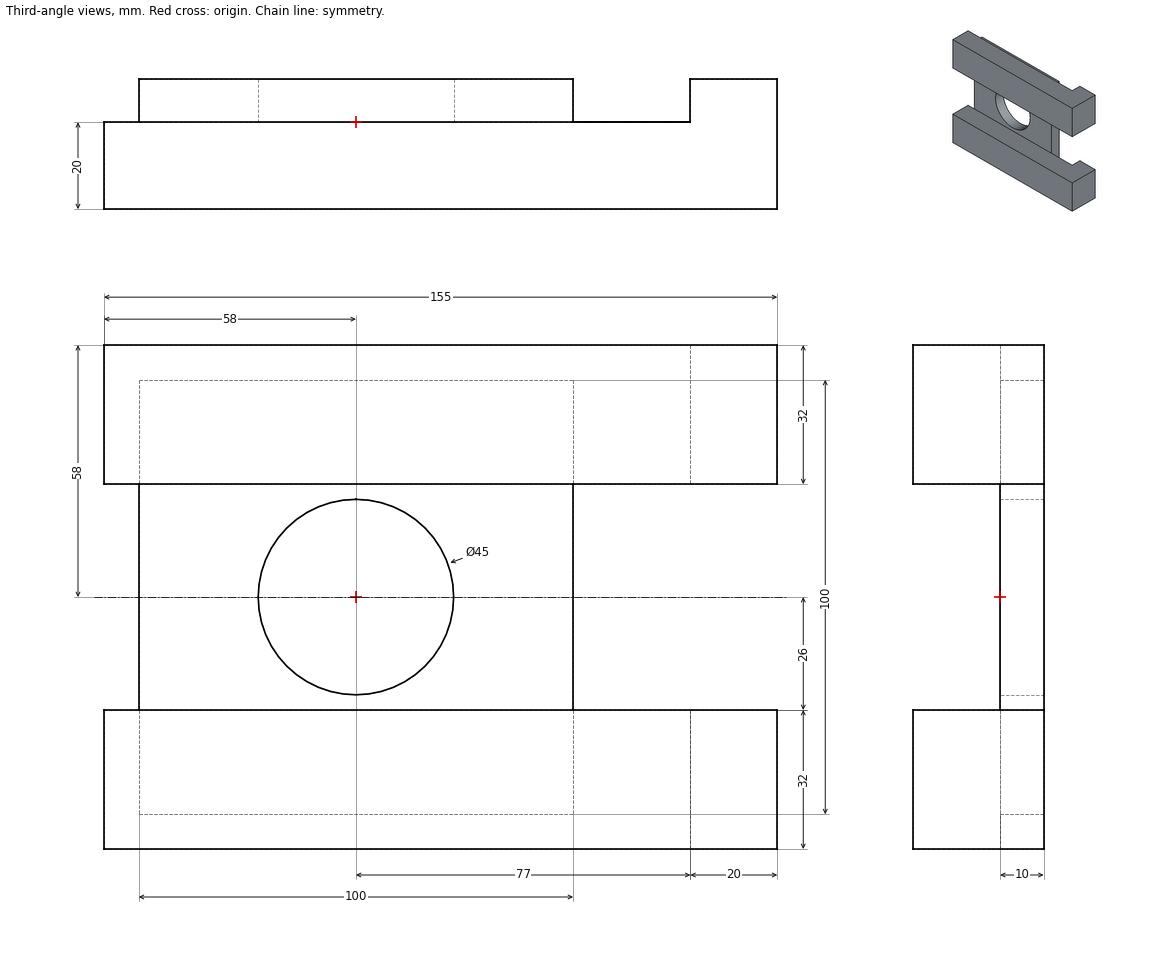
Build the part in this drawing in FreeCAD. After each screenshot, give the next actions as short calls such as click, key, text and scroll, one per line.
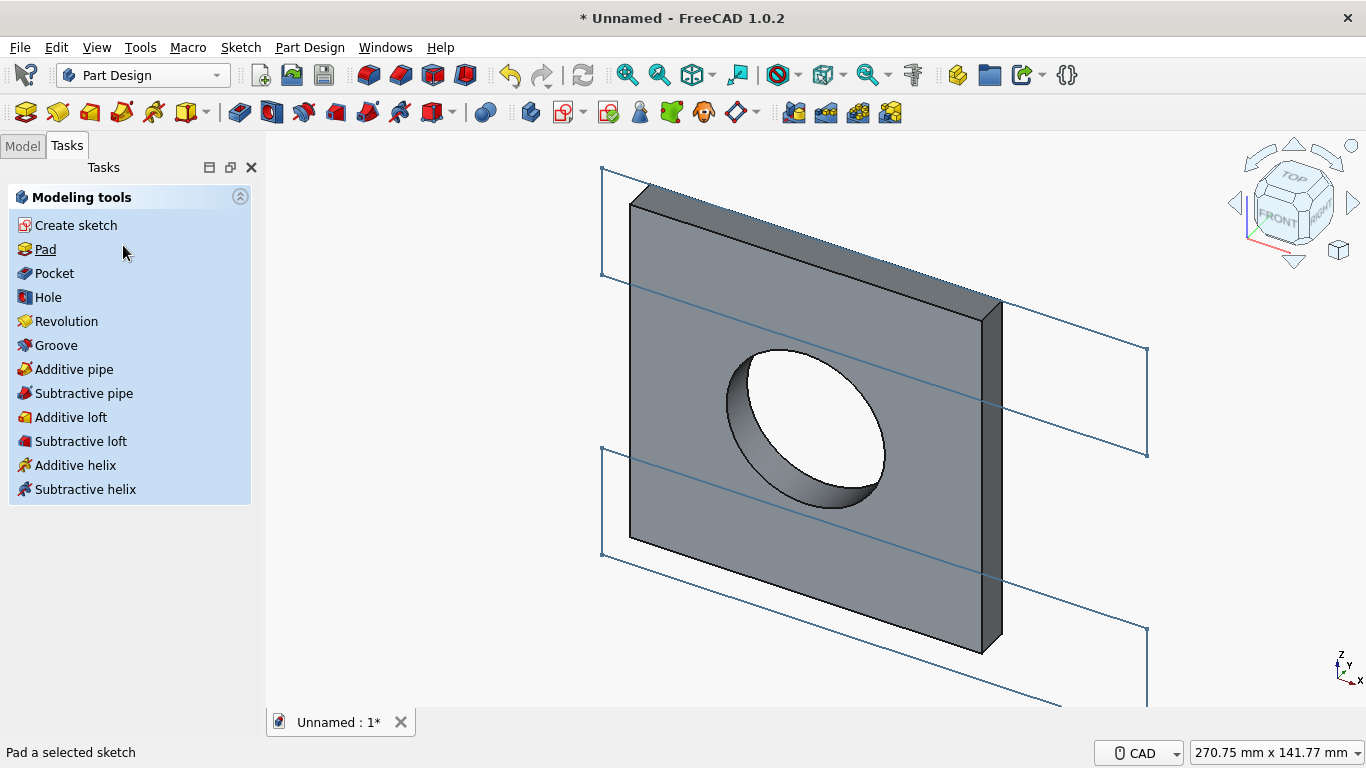
click(26, 112)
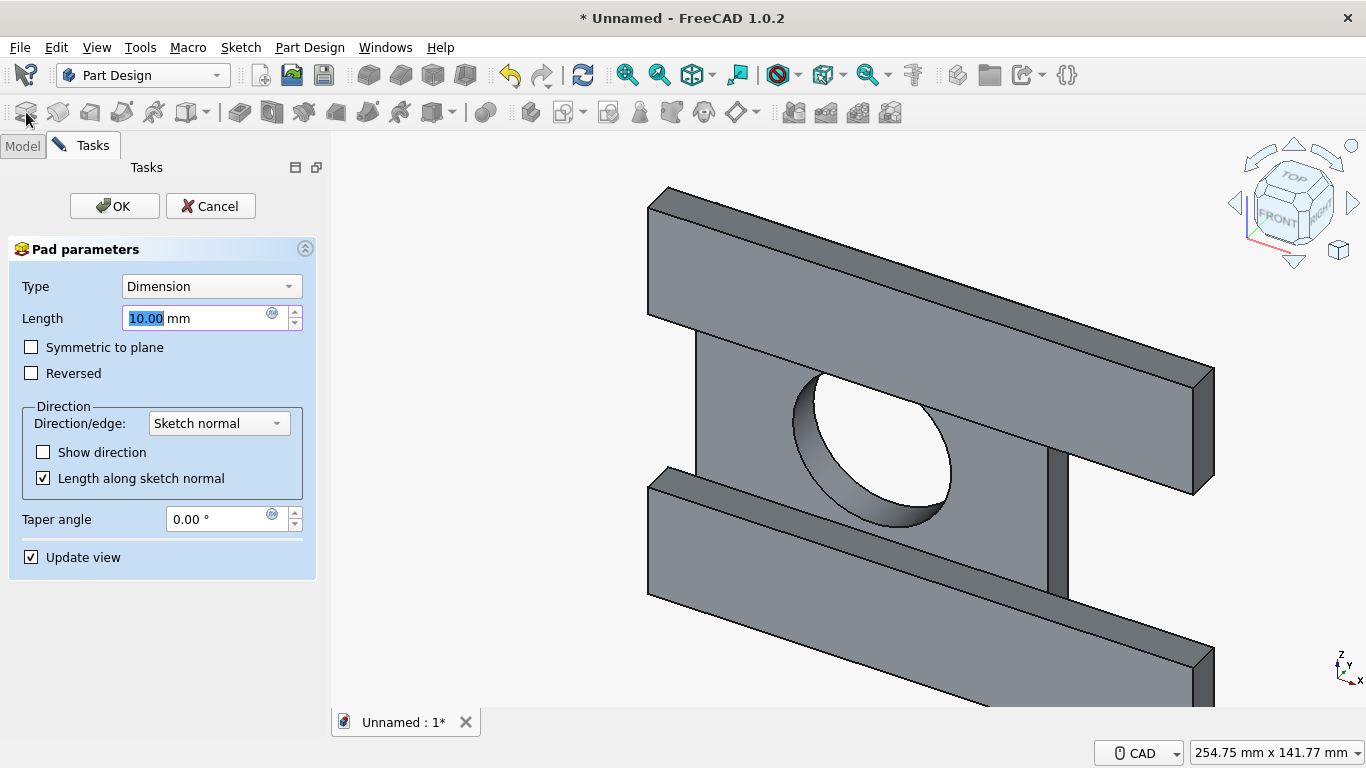
text(20)
key(Tab)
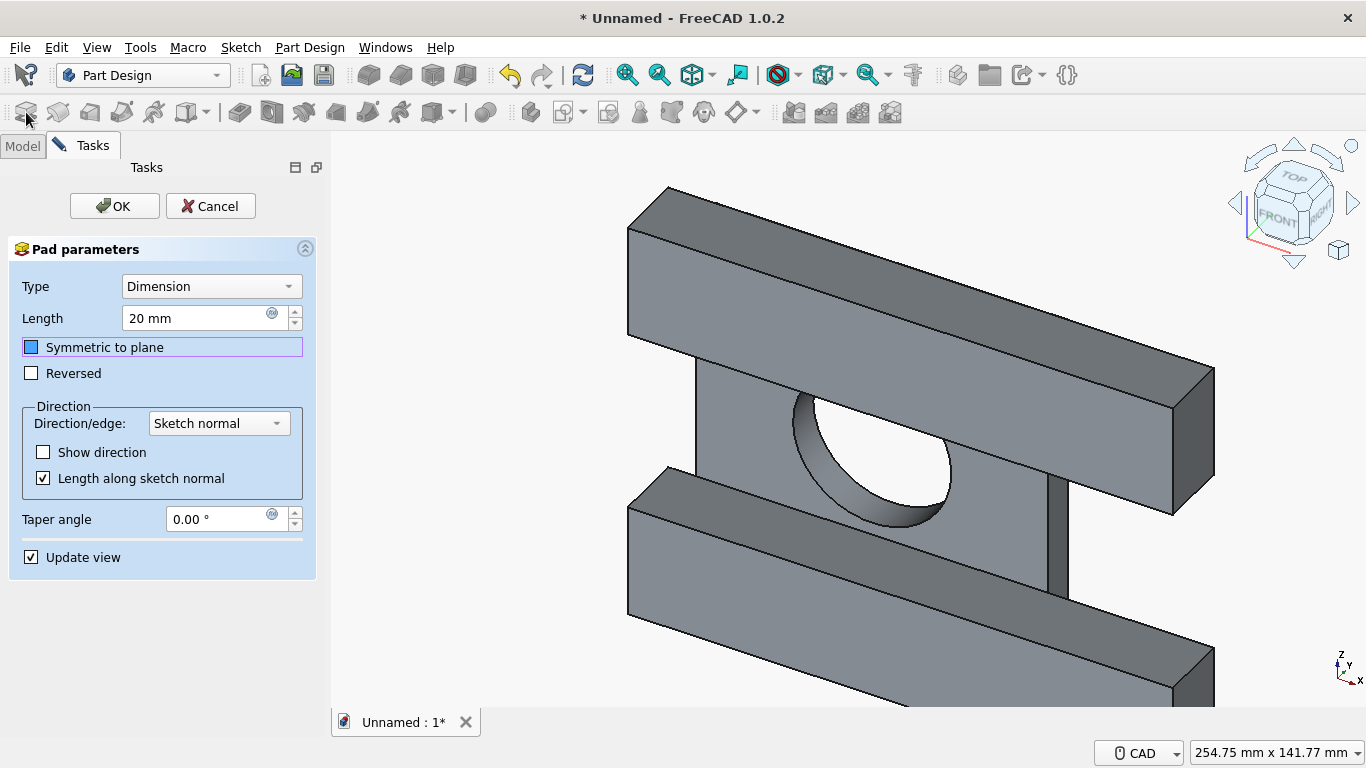
click(115, 206)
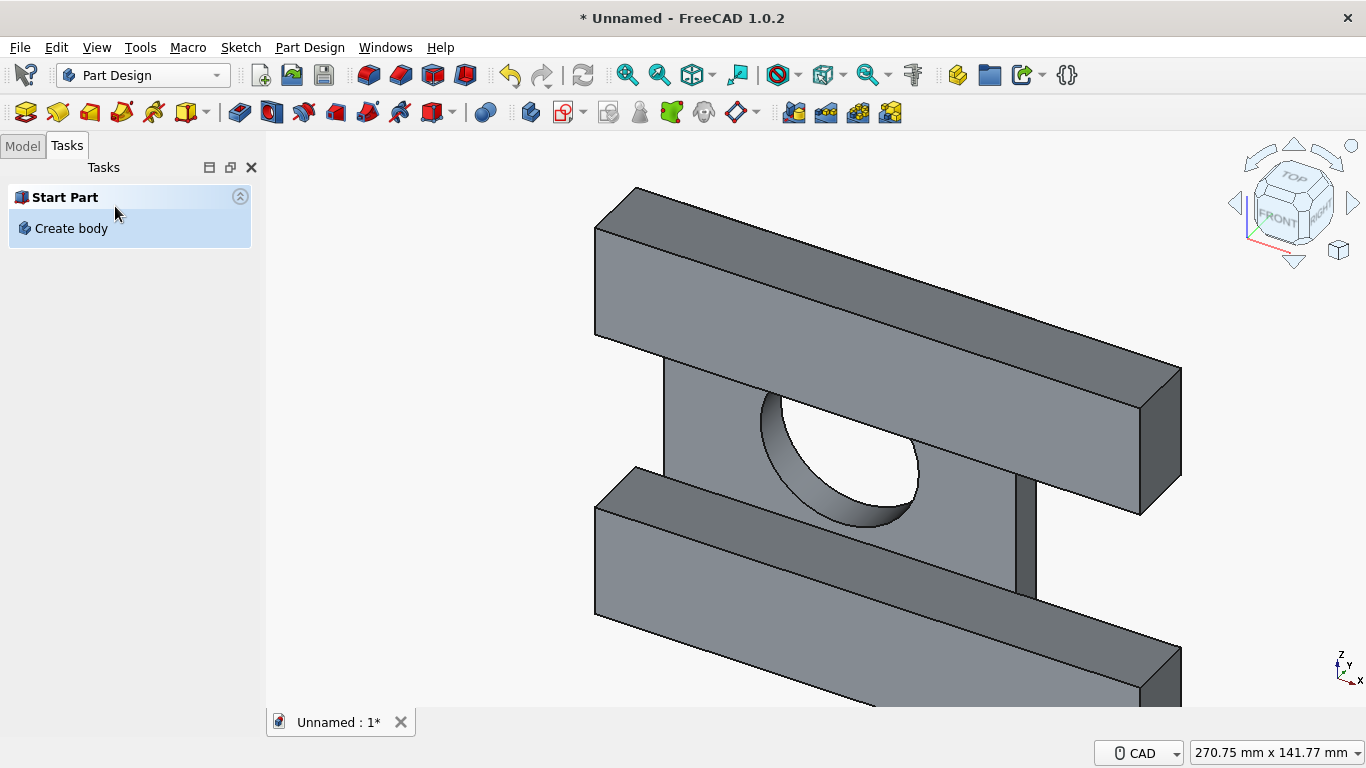
click(628, 76)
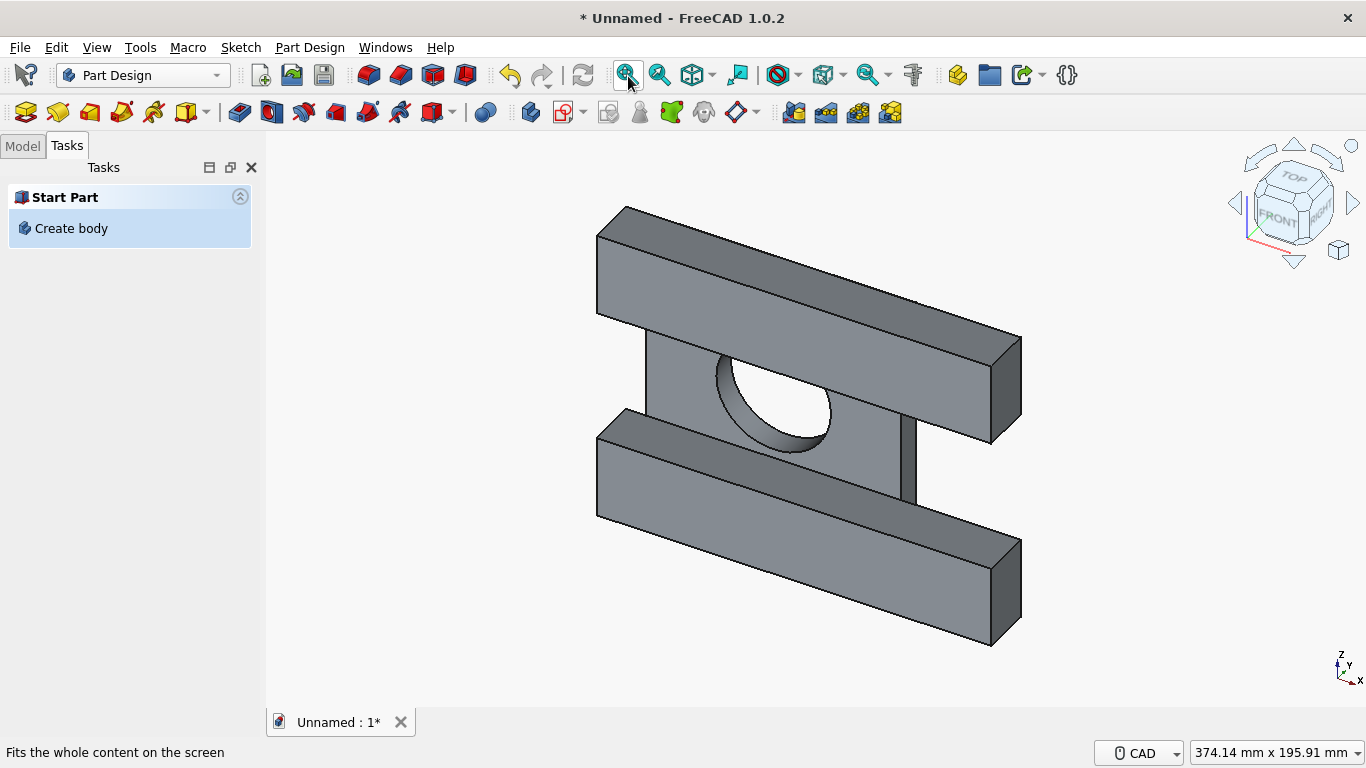
click(564, 112)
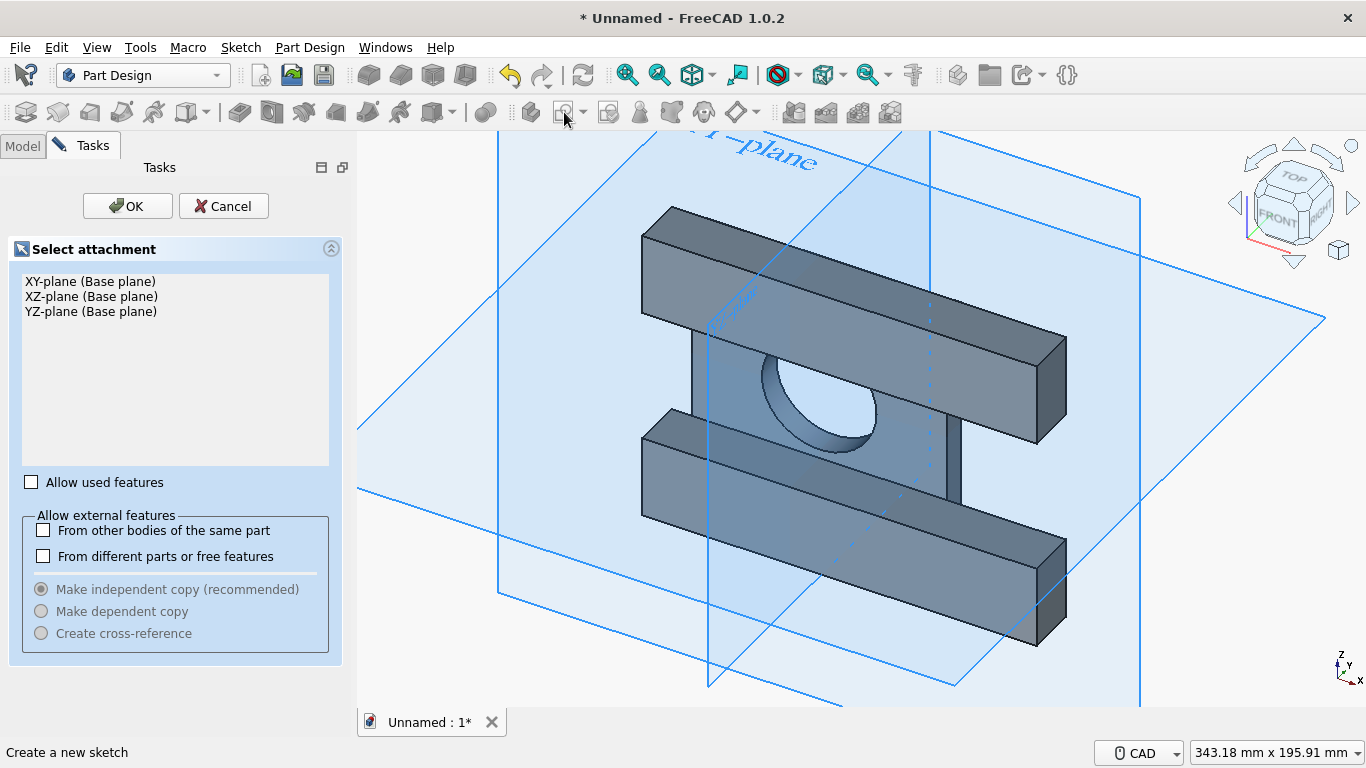
click(82, 296)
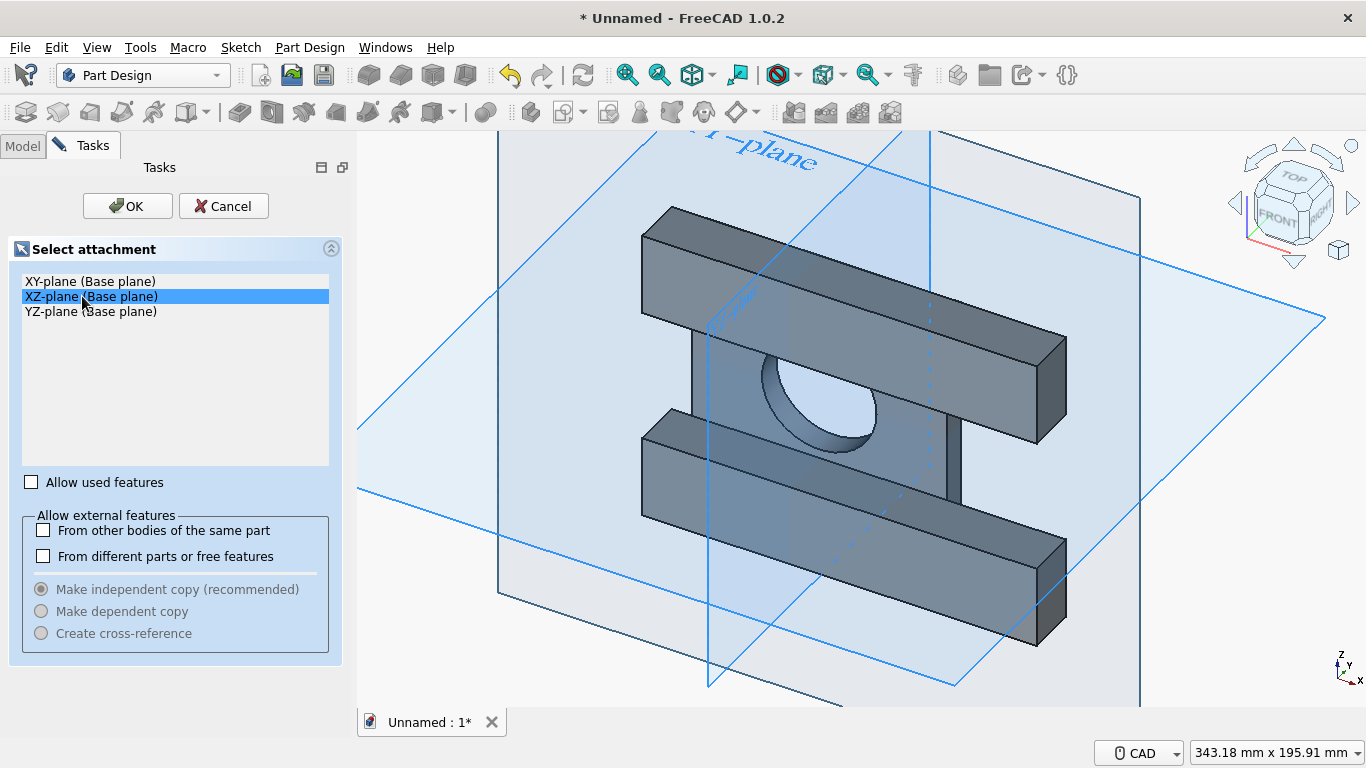
click(128, 206)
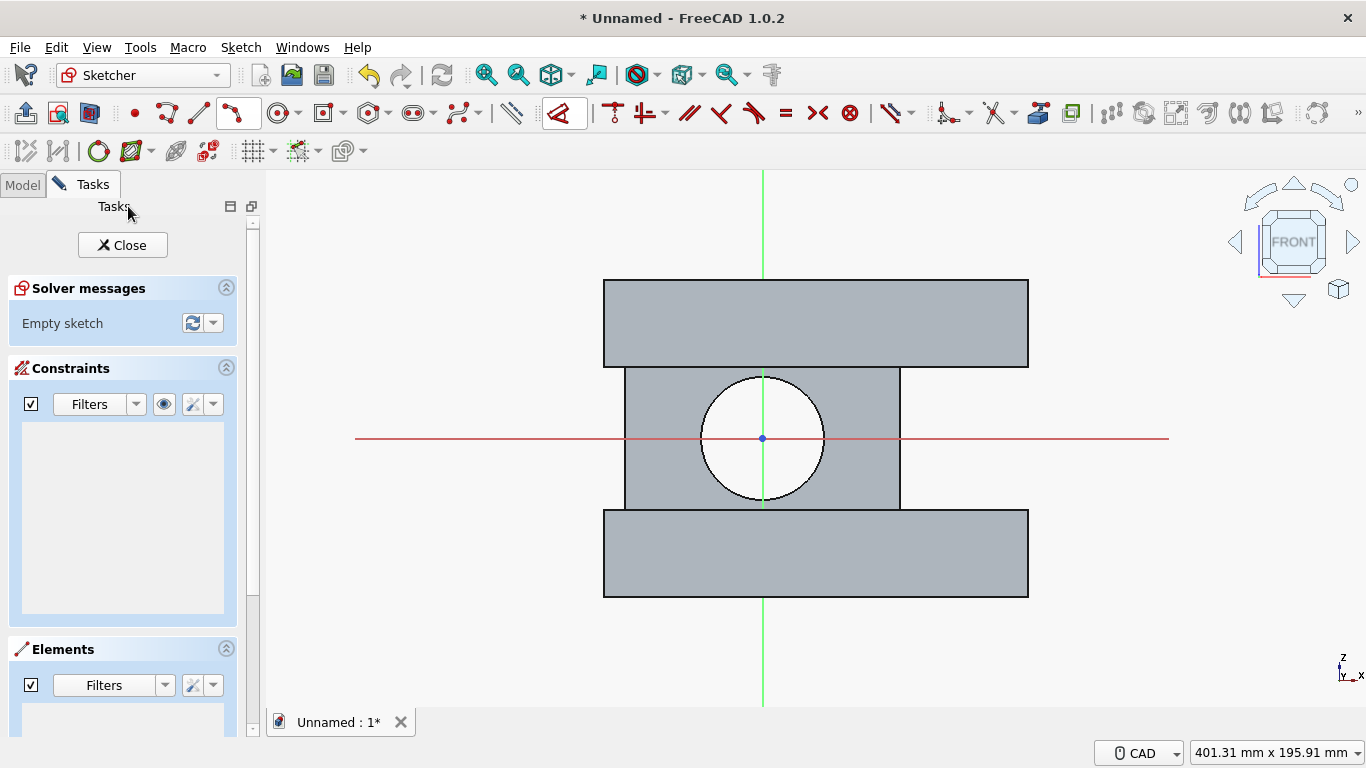
key(q)
key(s)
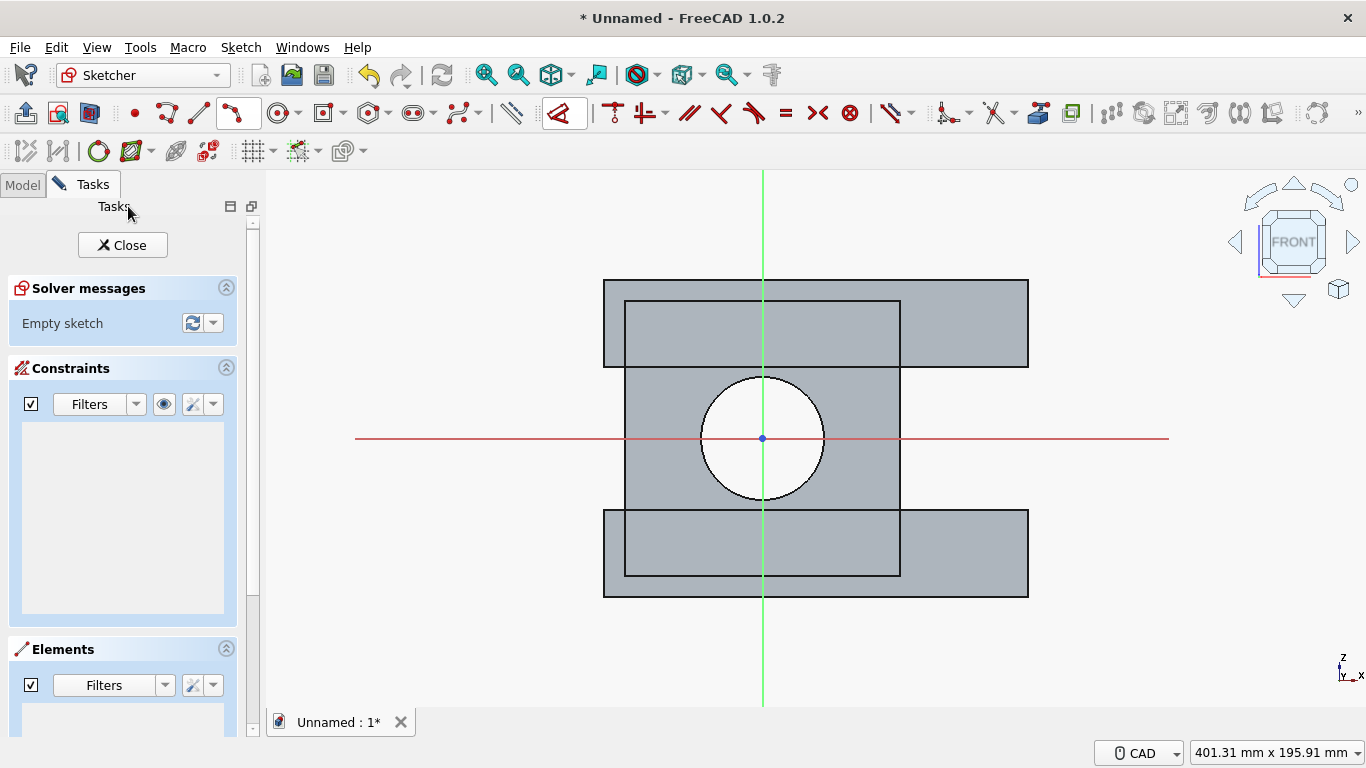
key(g)
key(r)